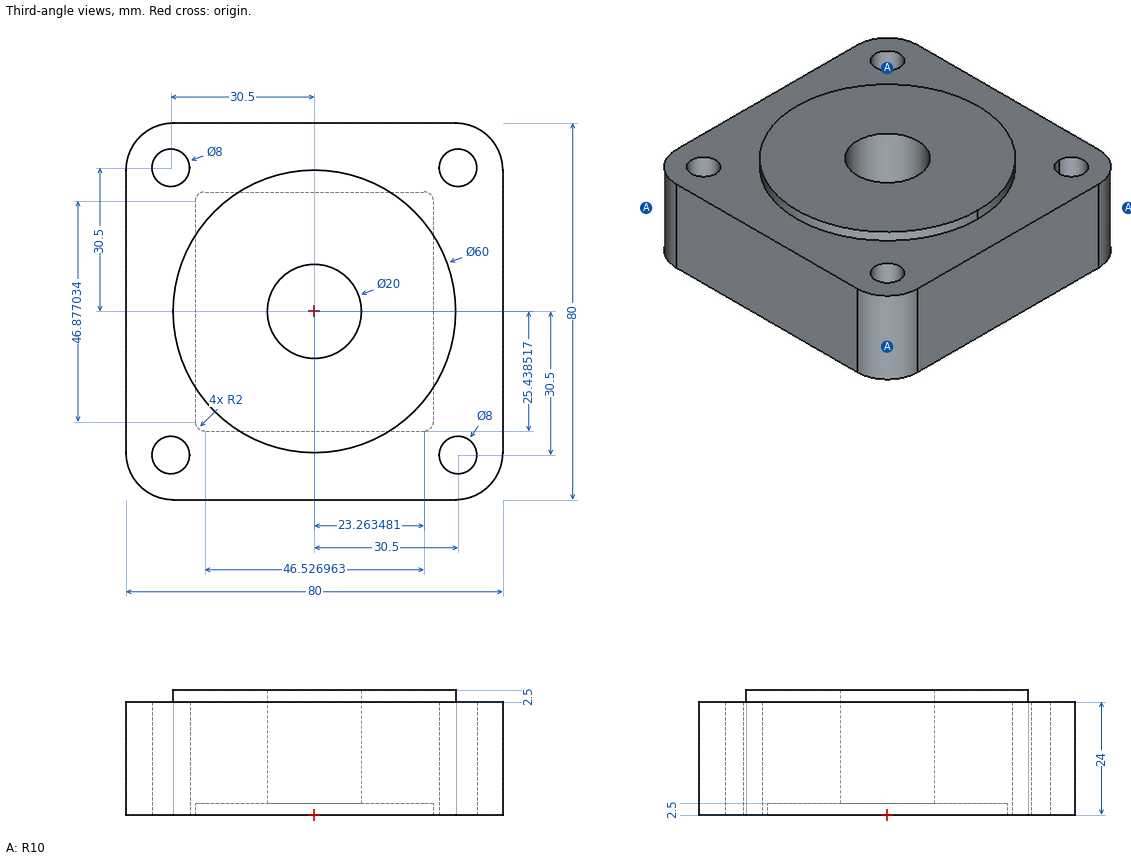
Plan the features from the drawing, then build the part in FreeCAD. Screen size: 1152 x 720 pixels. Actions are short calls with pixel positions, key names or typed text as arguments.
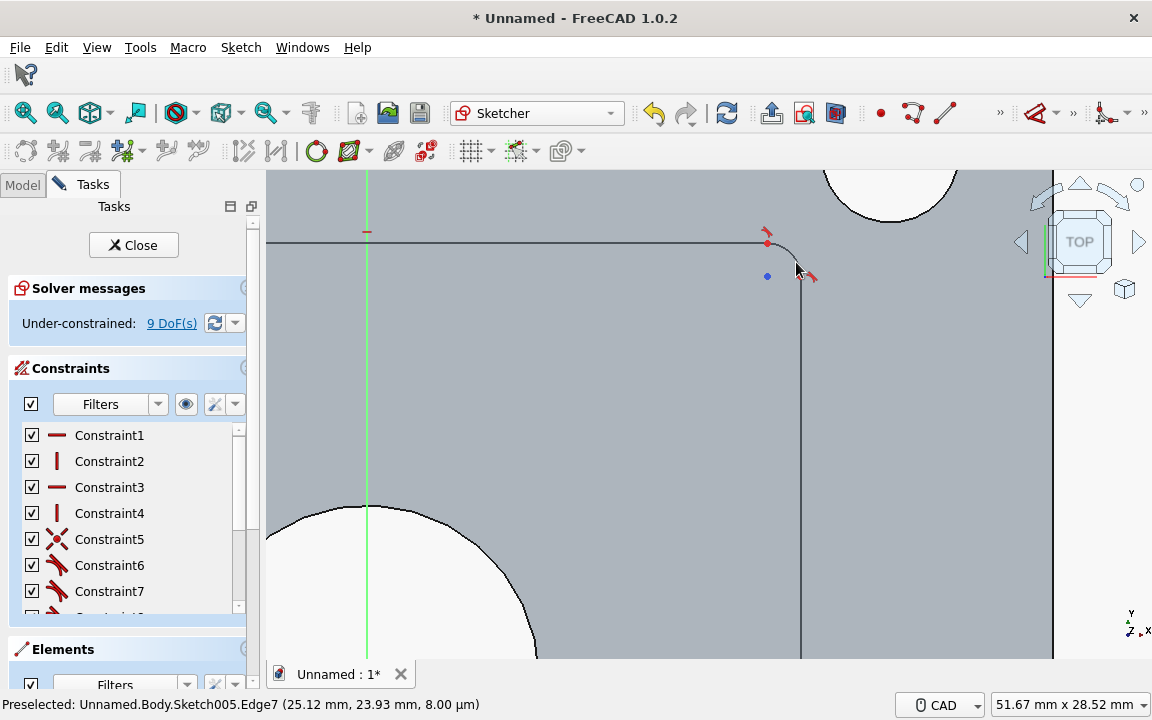
click(801, 518)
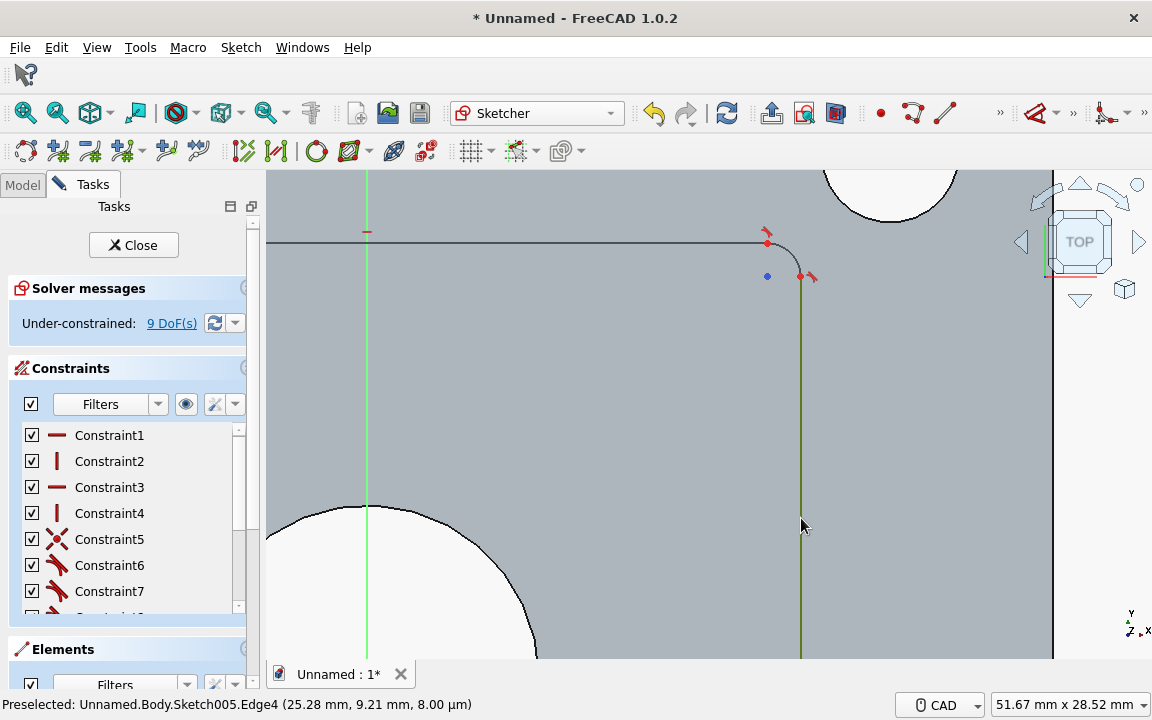
scroll(800, 262, down, 5)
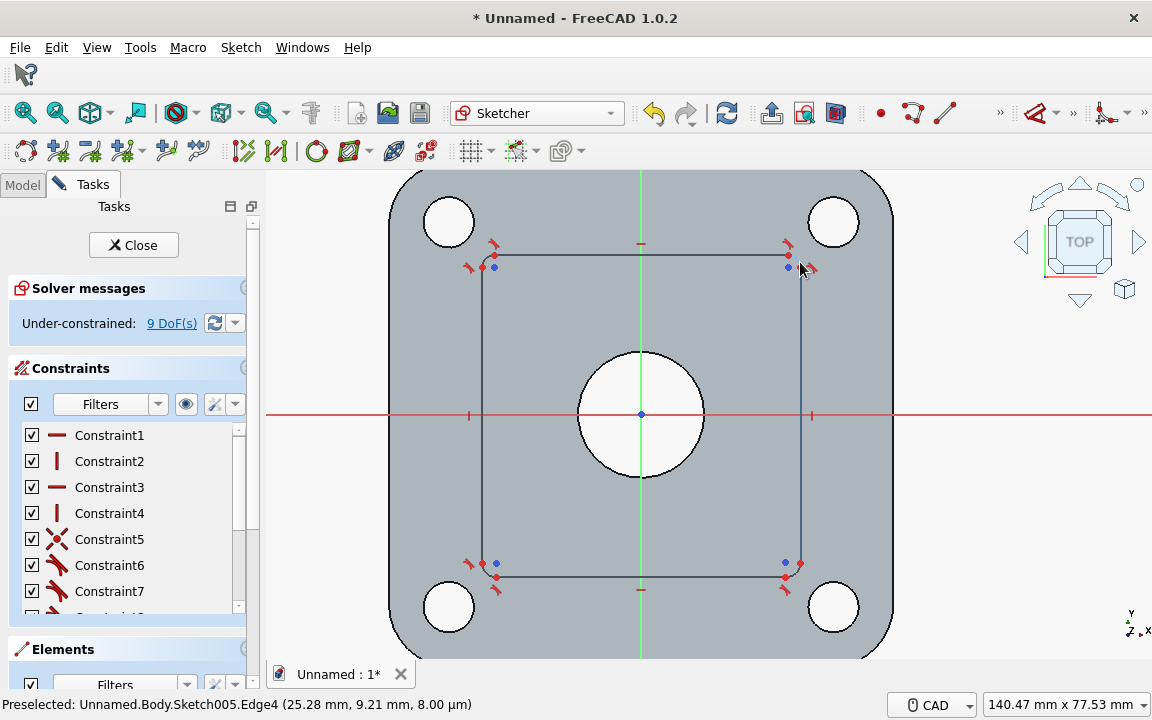
scroll(792, 576, up, 4)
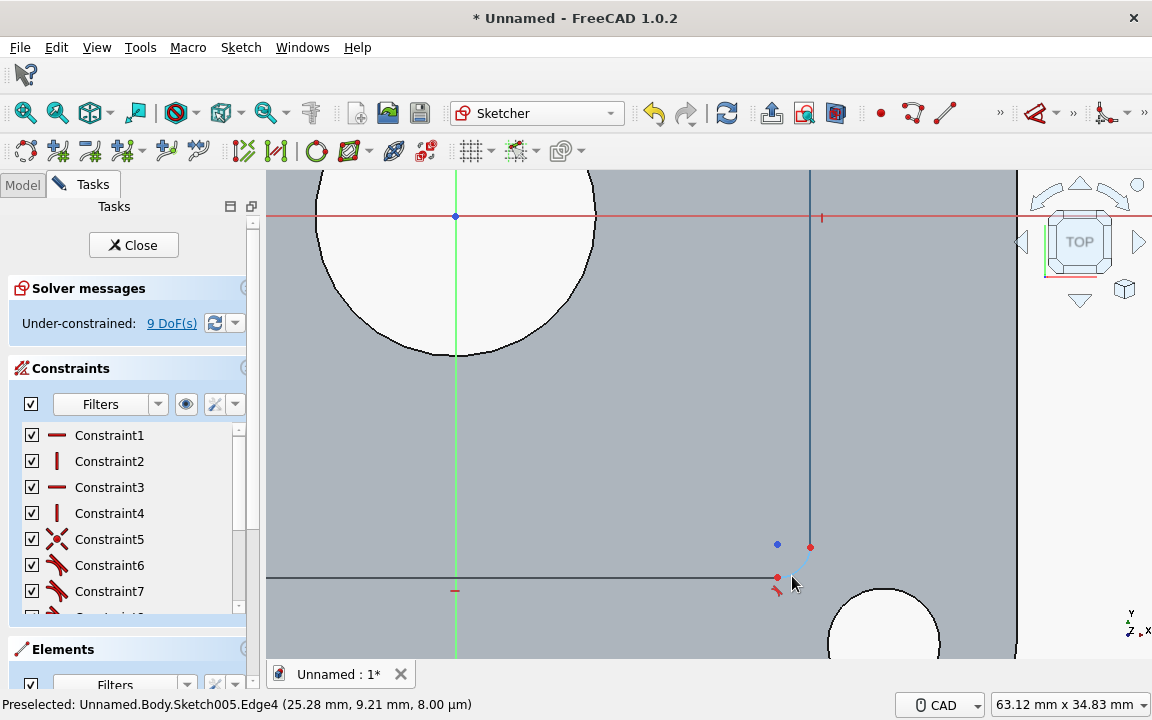
click(792, 575)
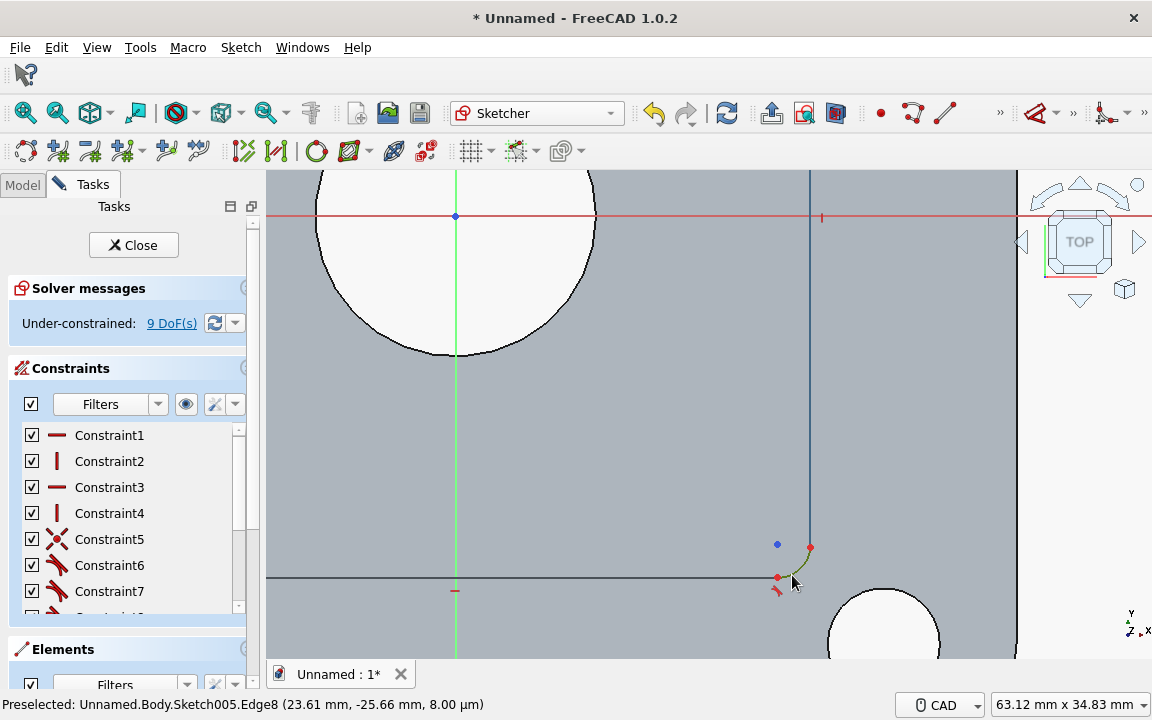
key(t)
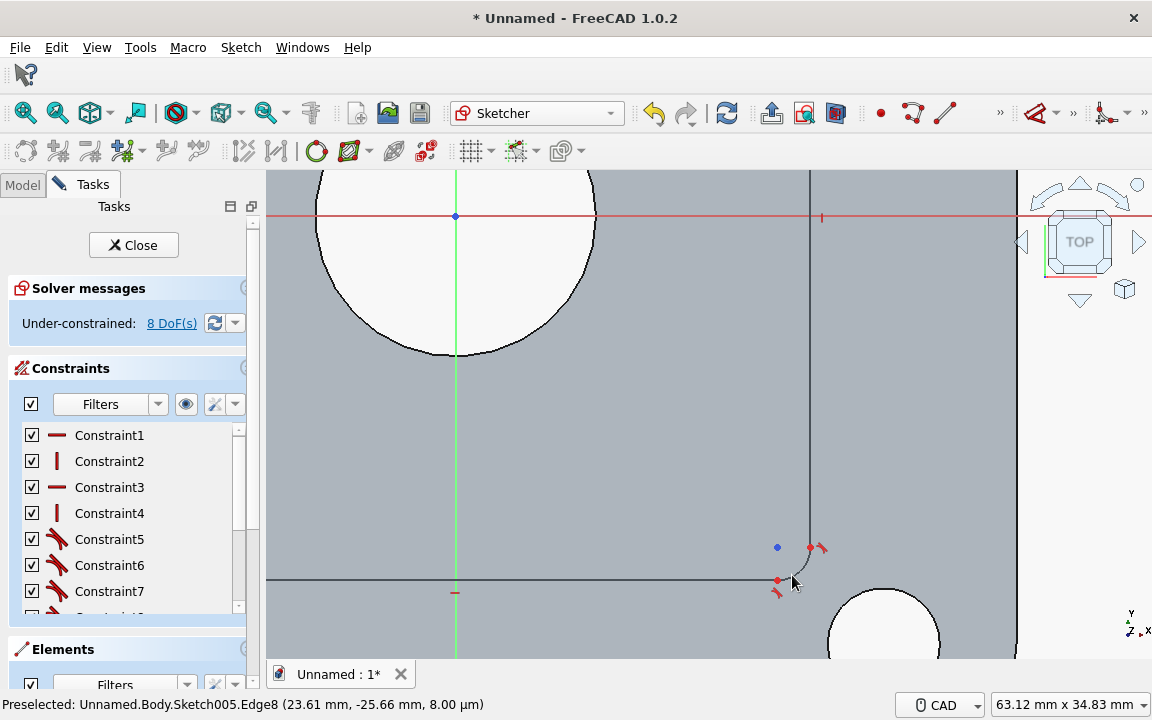
scroll(791, 576, down, 4)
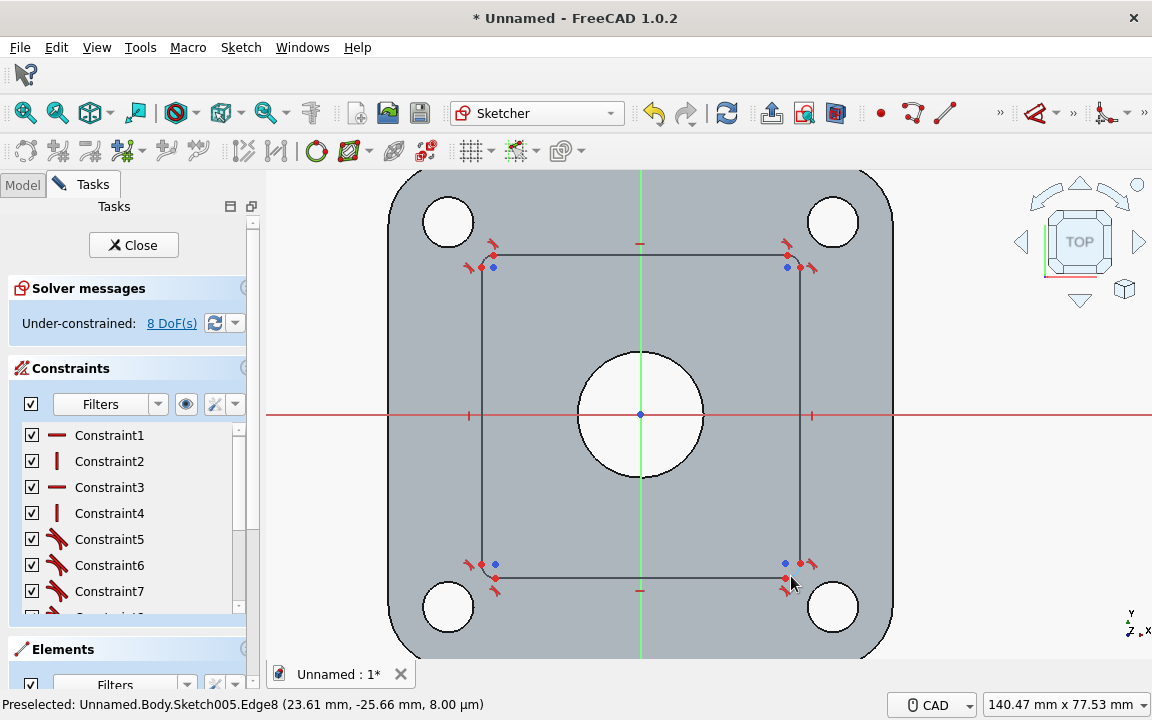
scroll(483, 571, up, 4)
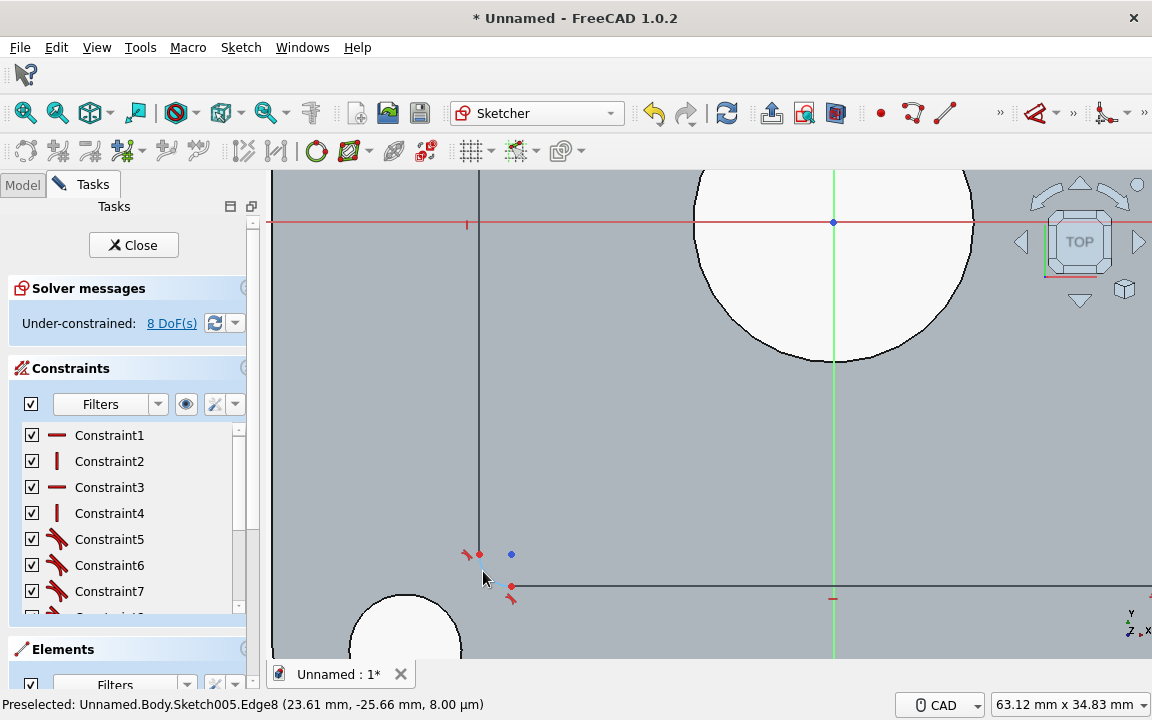
click(483, 569)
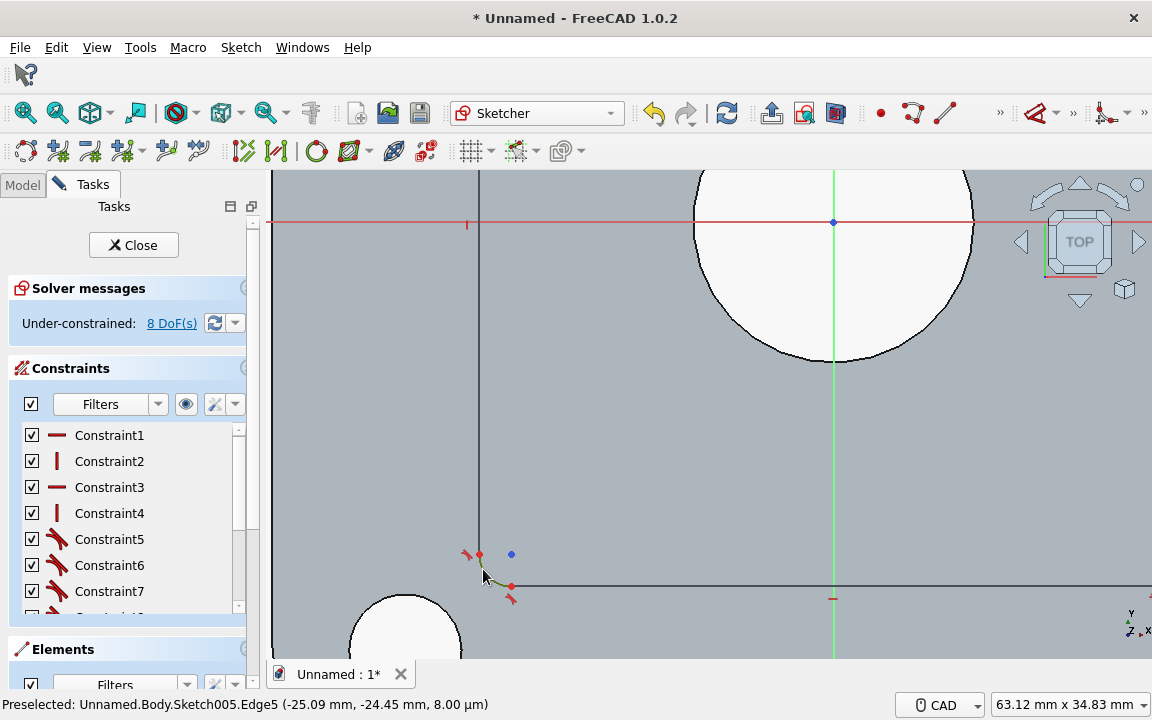
scroll(483, 571, down, 4)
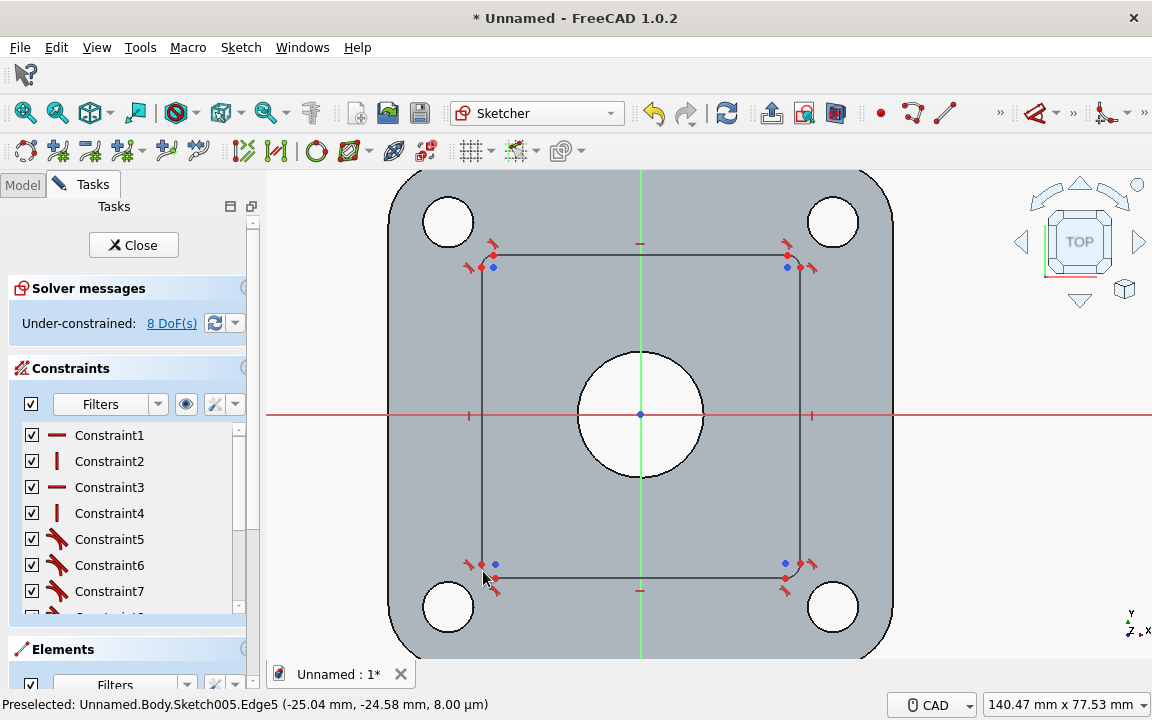
scroll(488, 257, up, 5)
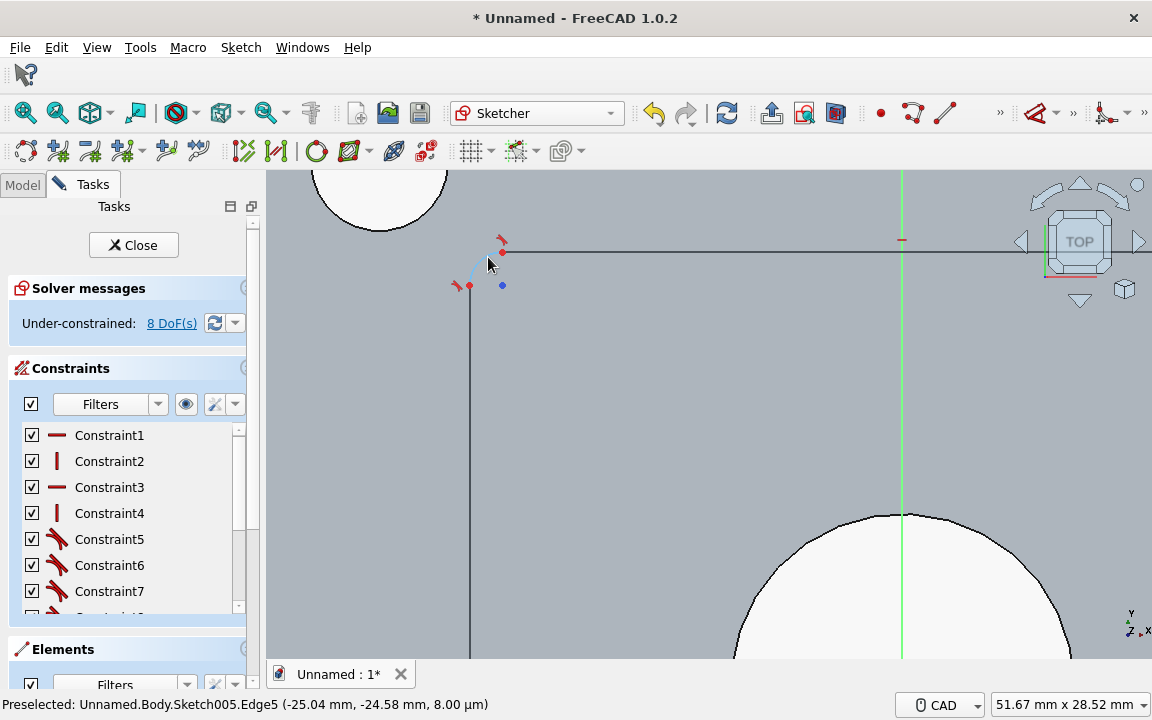
click(488, 256)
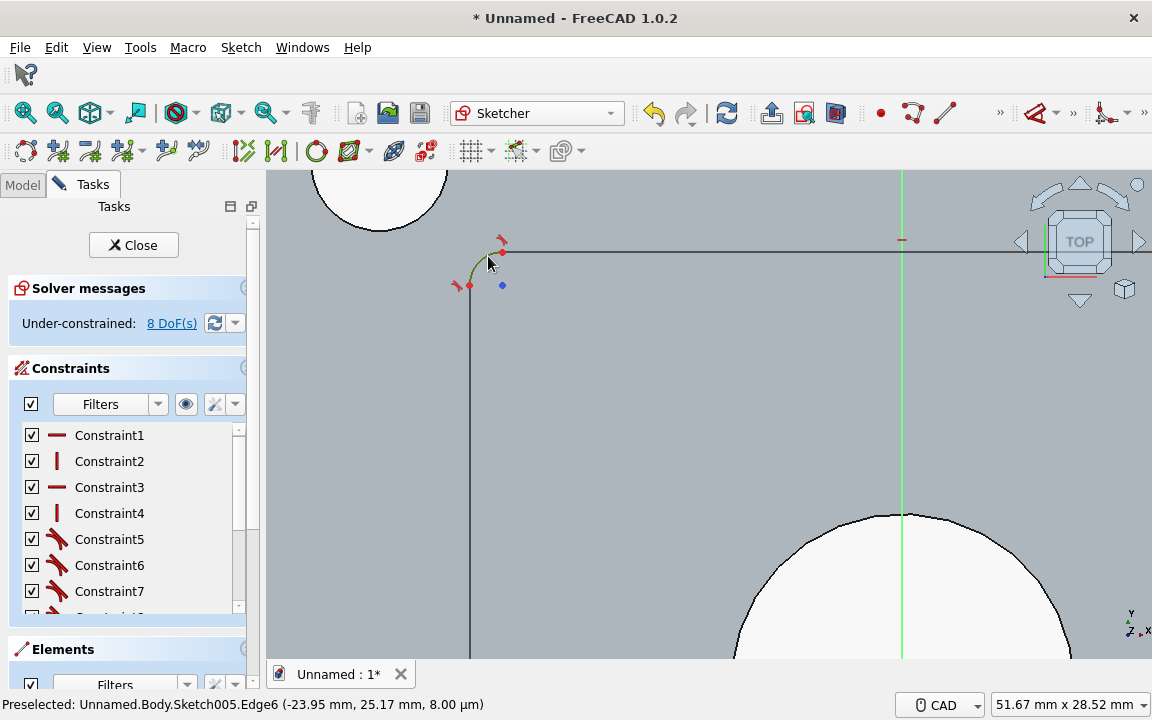
scroll(488, 257, down, 5)